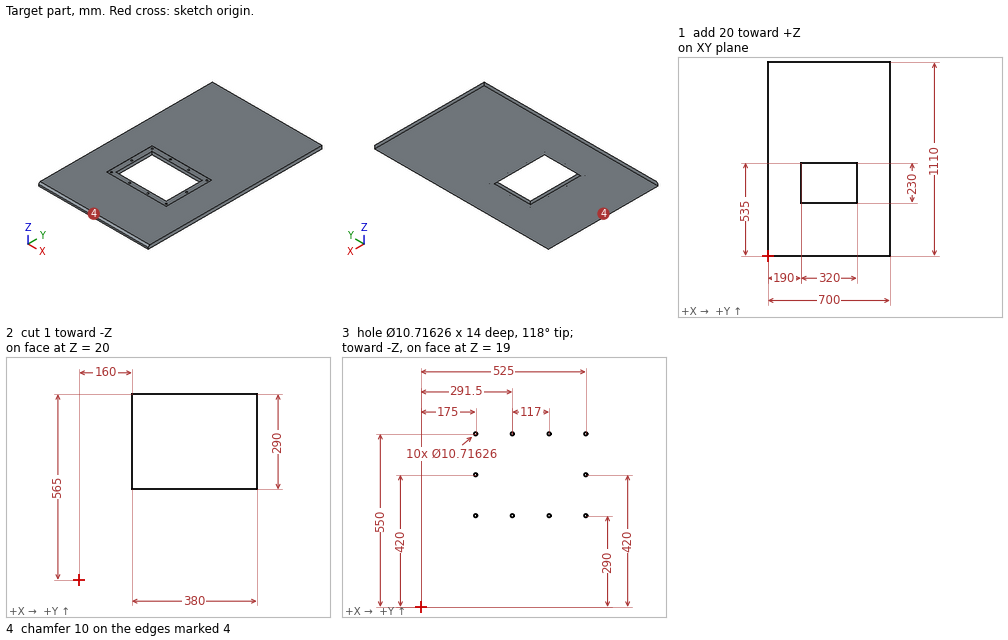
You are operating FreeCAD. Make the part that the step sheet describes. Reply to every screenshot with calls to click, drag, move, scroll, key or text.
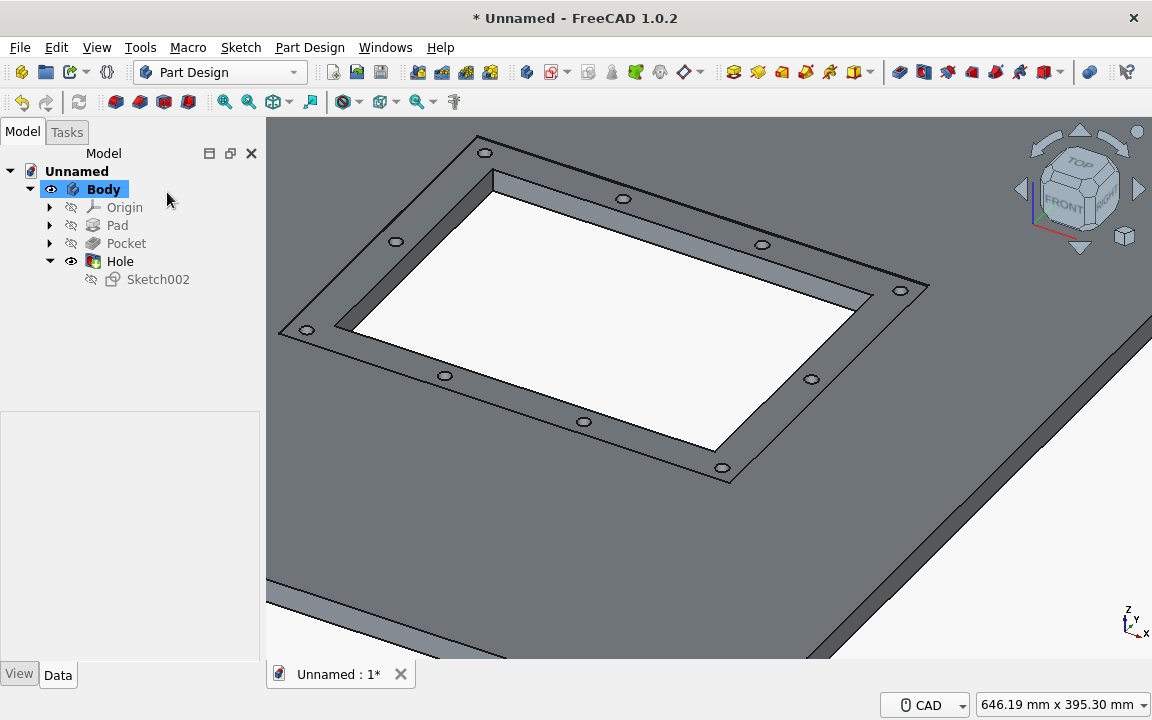
click(226, 102)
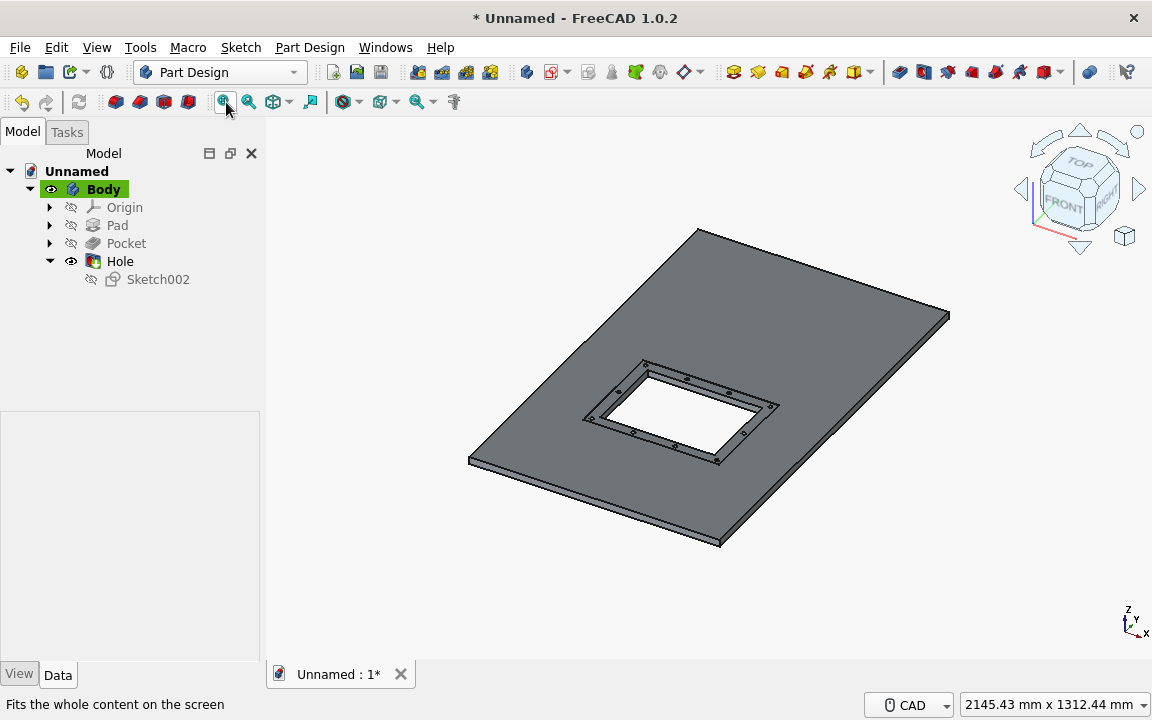
click(594, 497)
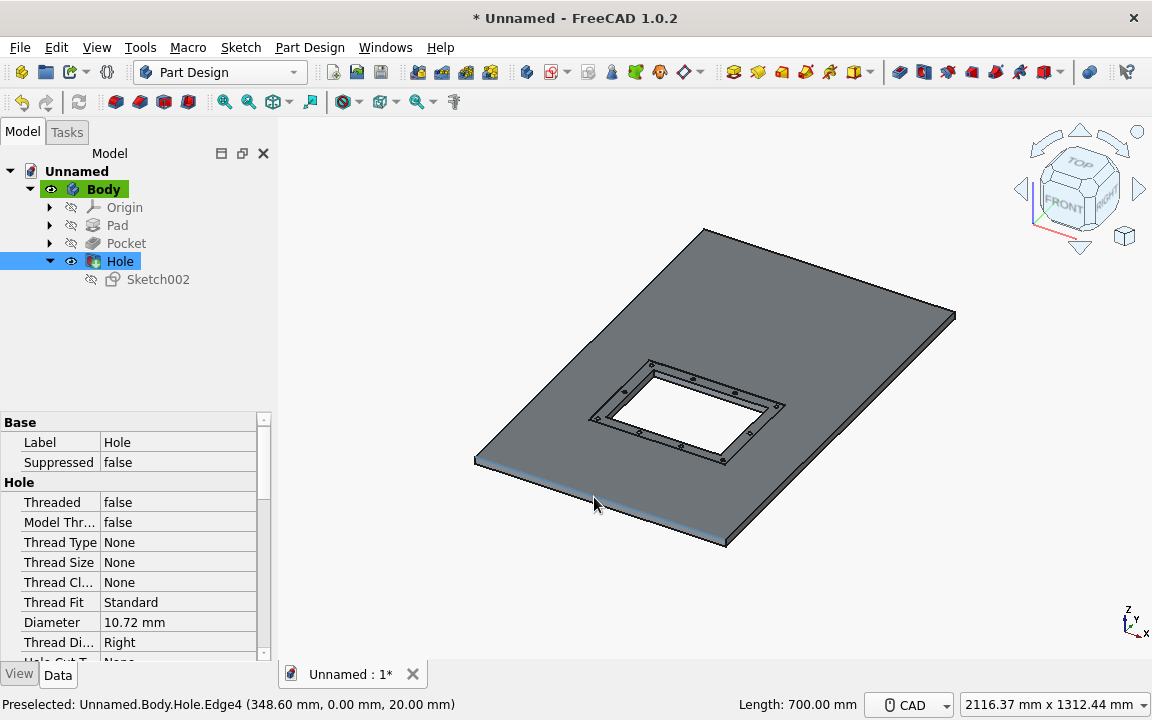
click(140, 102)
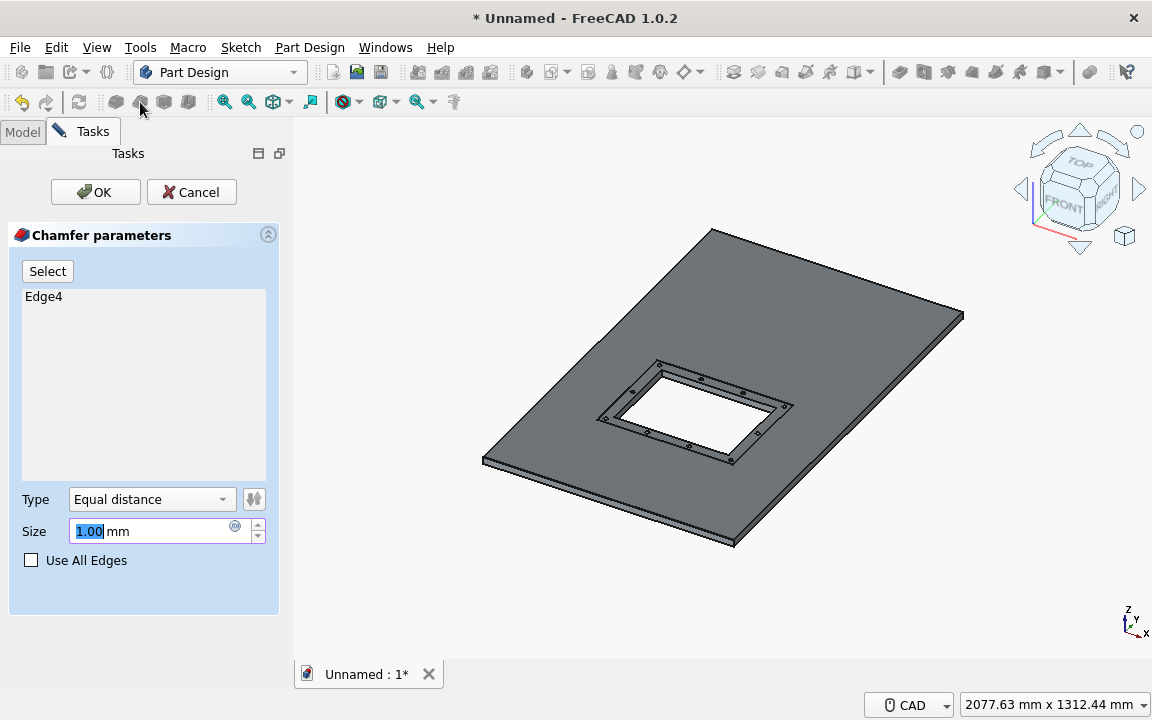
text(10)
key(Tab)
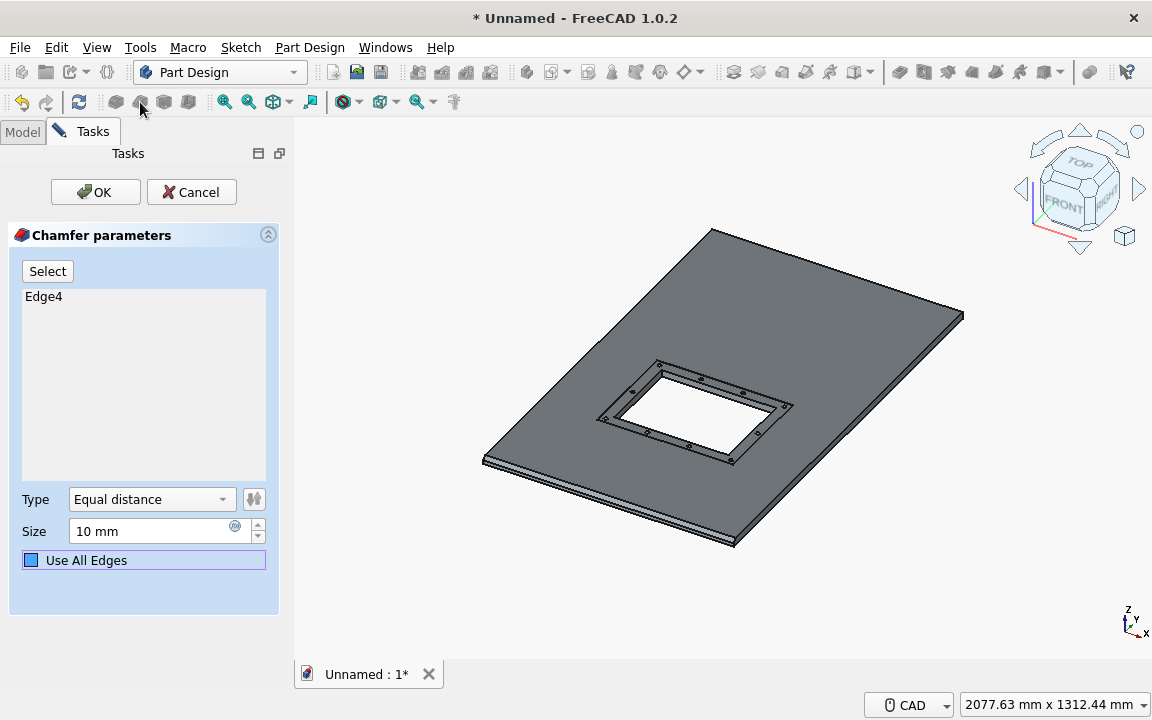
click(96, 192)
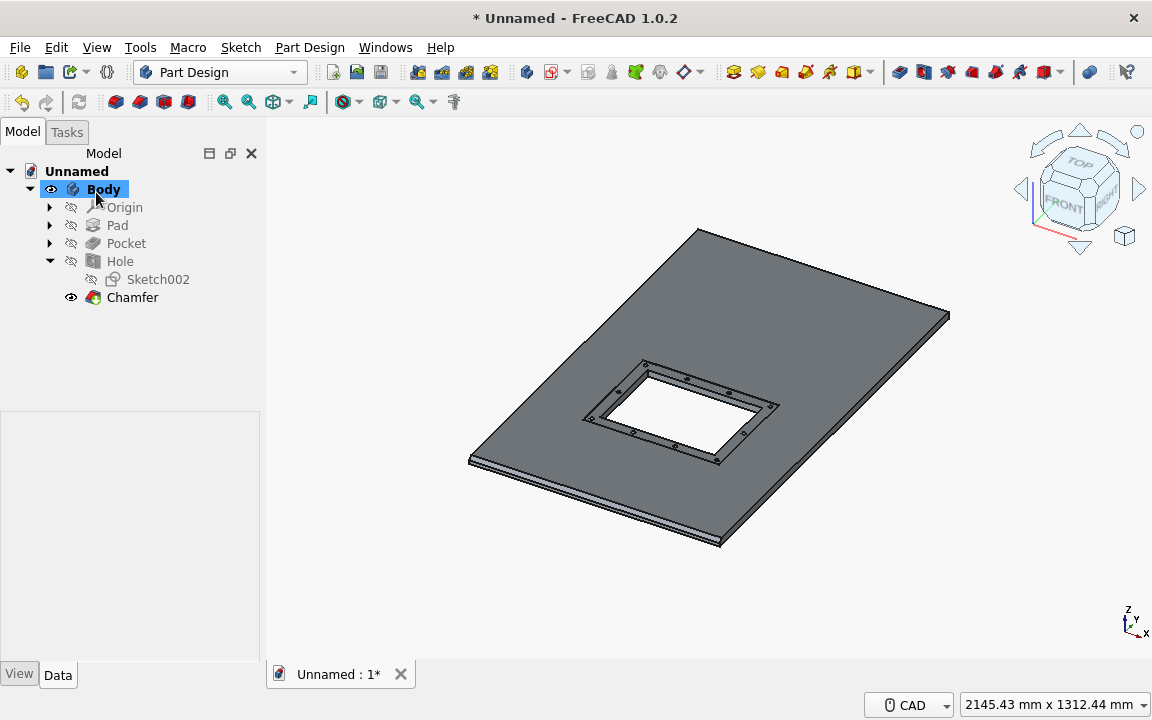
key(0)